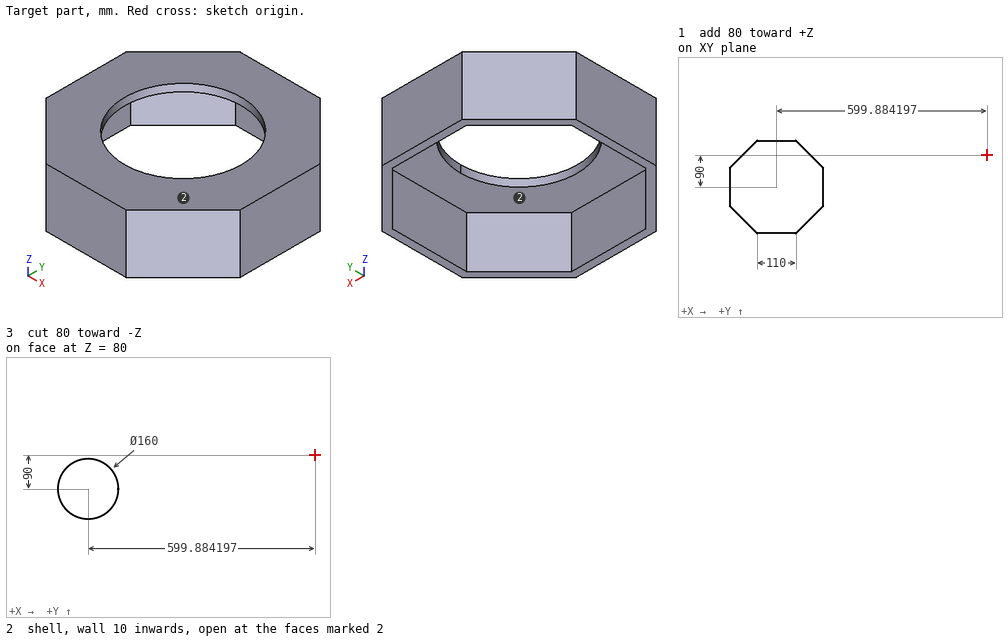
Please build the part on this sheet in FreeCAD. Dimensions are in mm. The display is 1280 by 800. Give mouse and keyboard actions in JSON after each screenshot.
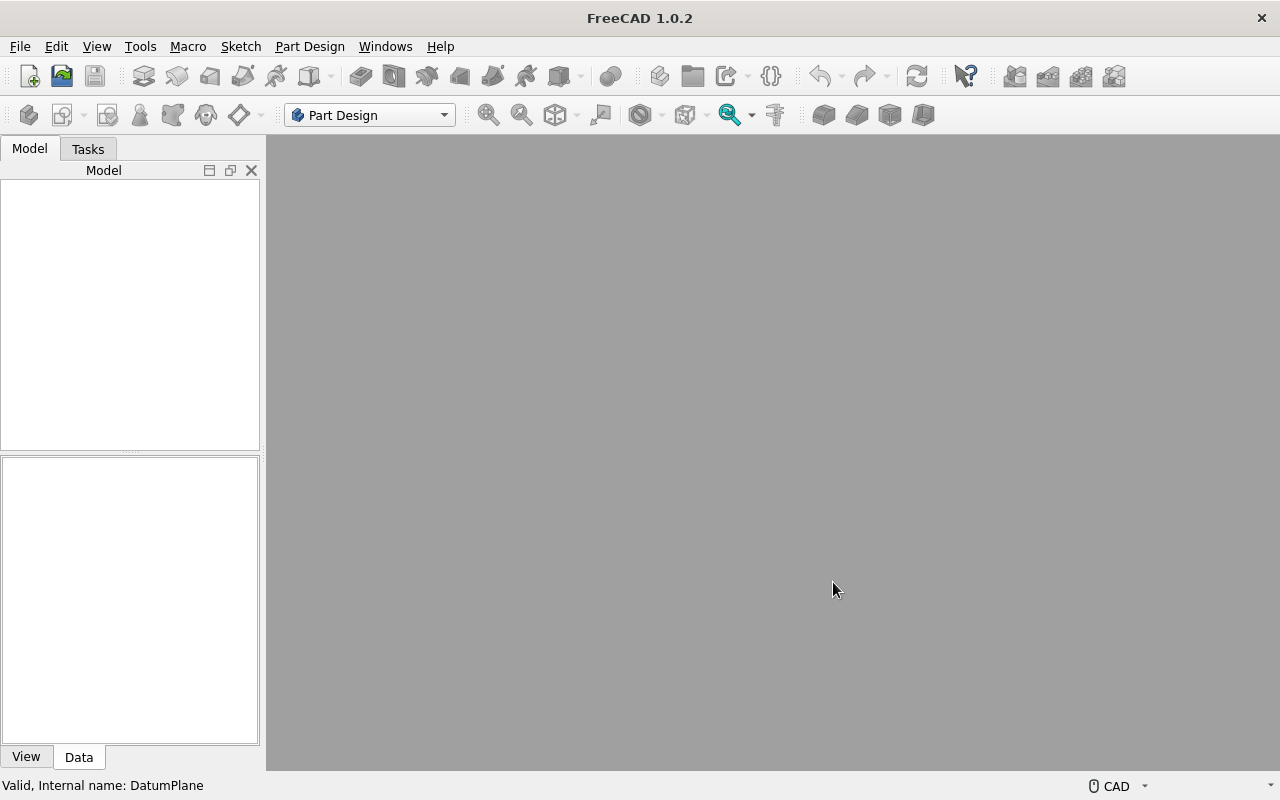
{"action": "key", "text": "ctrl+n"}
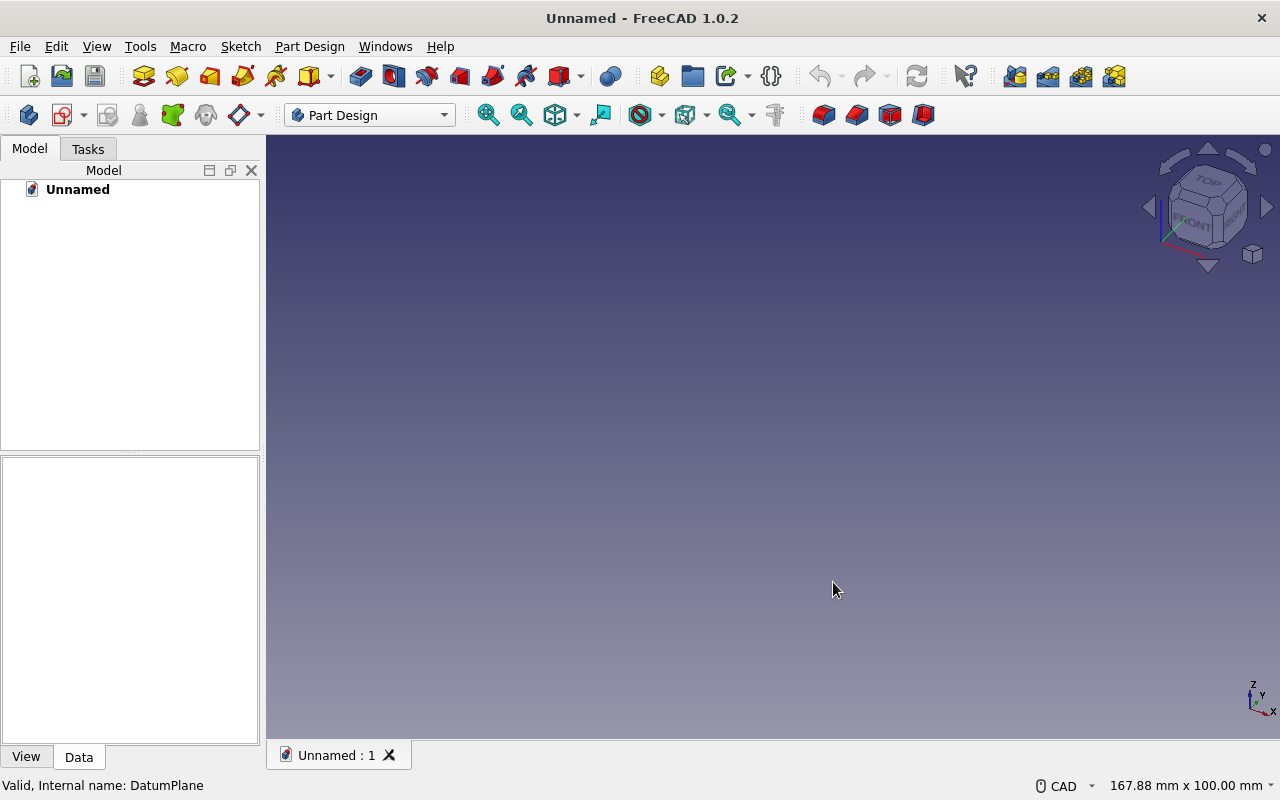
{"action": "left_click", "coordinate": [62, 116]}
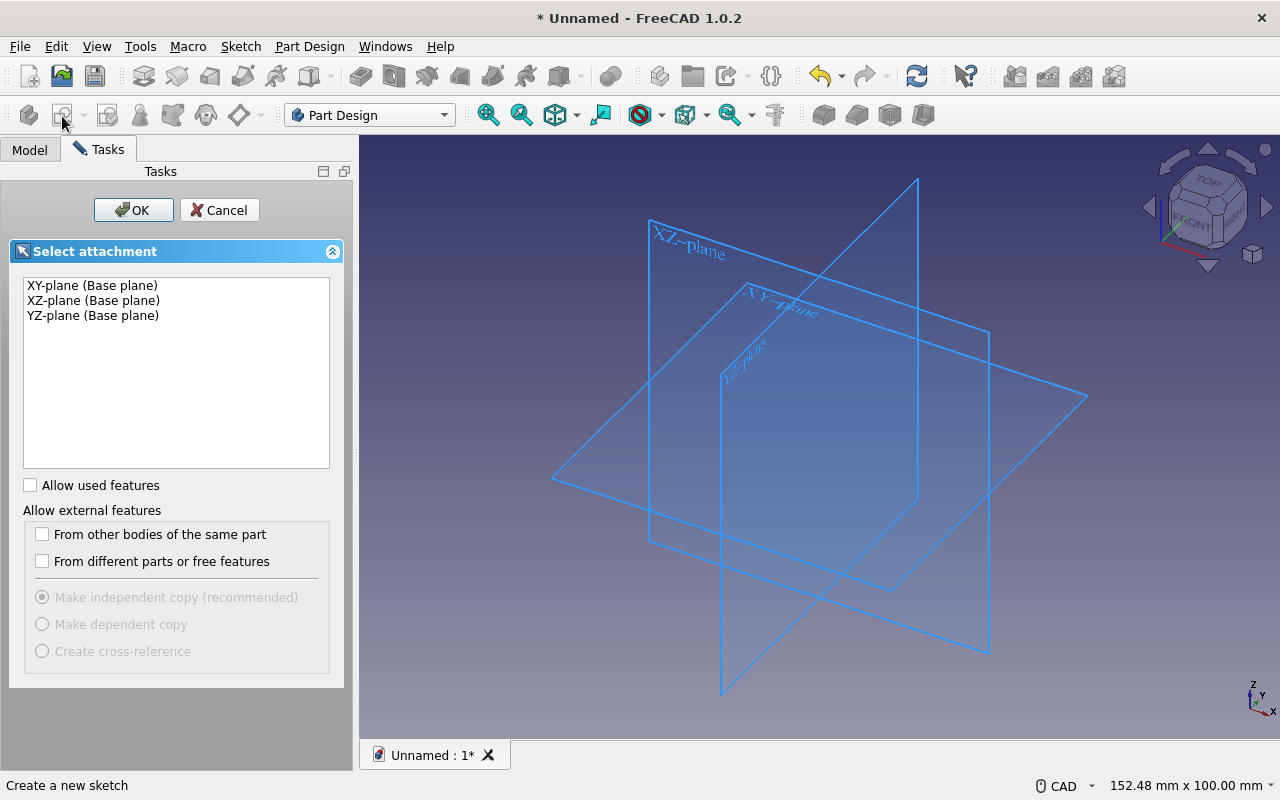
{"action": "left_click", "coordinate": [84, 286]}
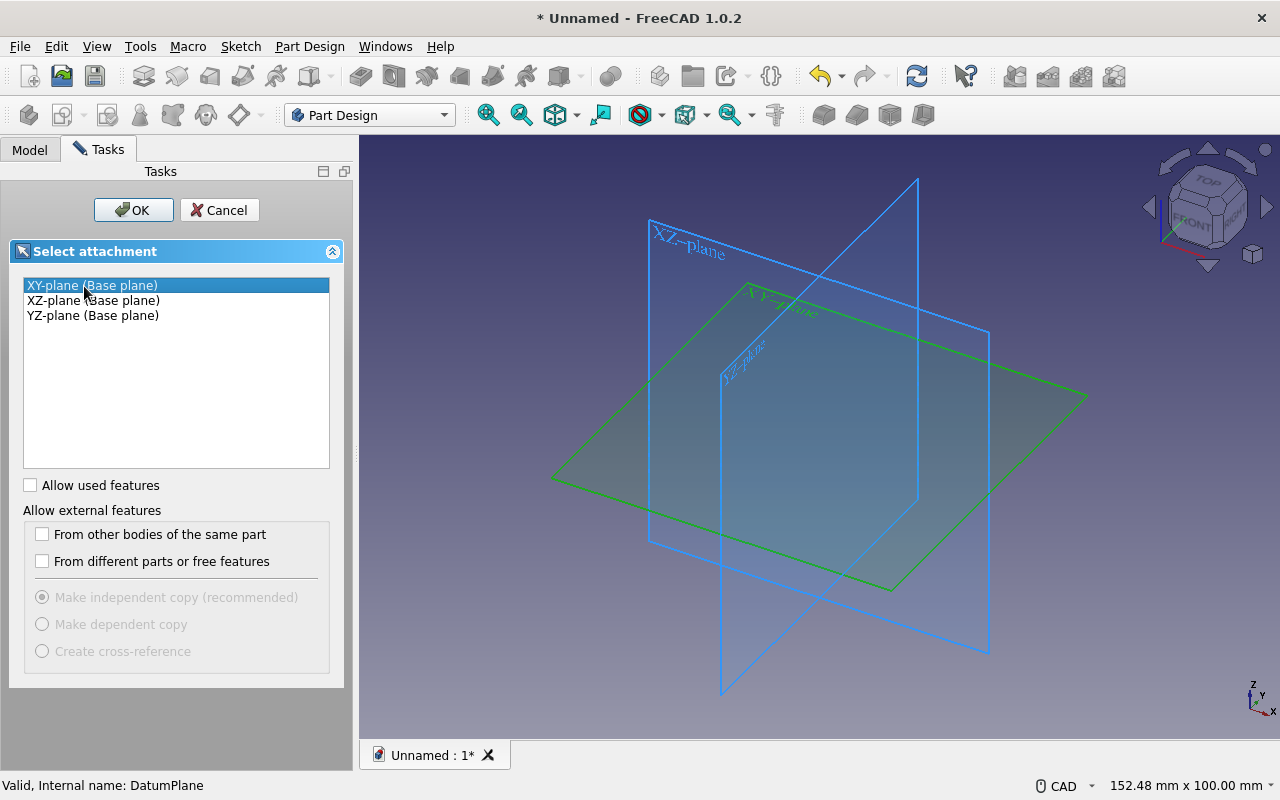
{"action": "left_click", "coordinate": [134, 210]}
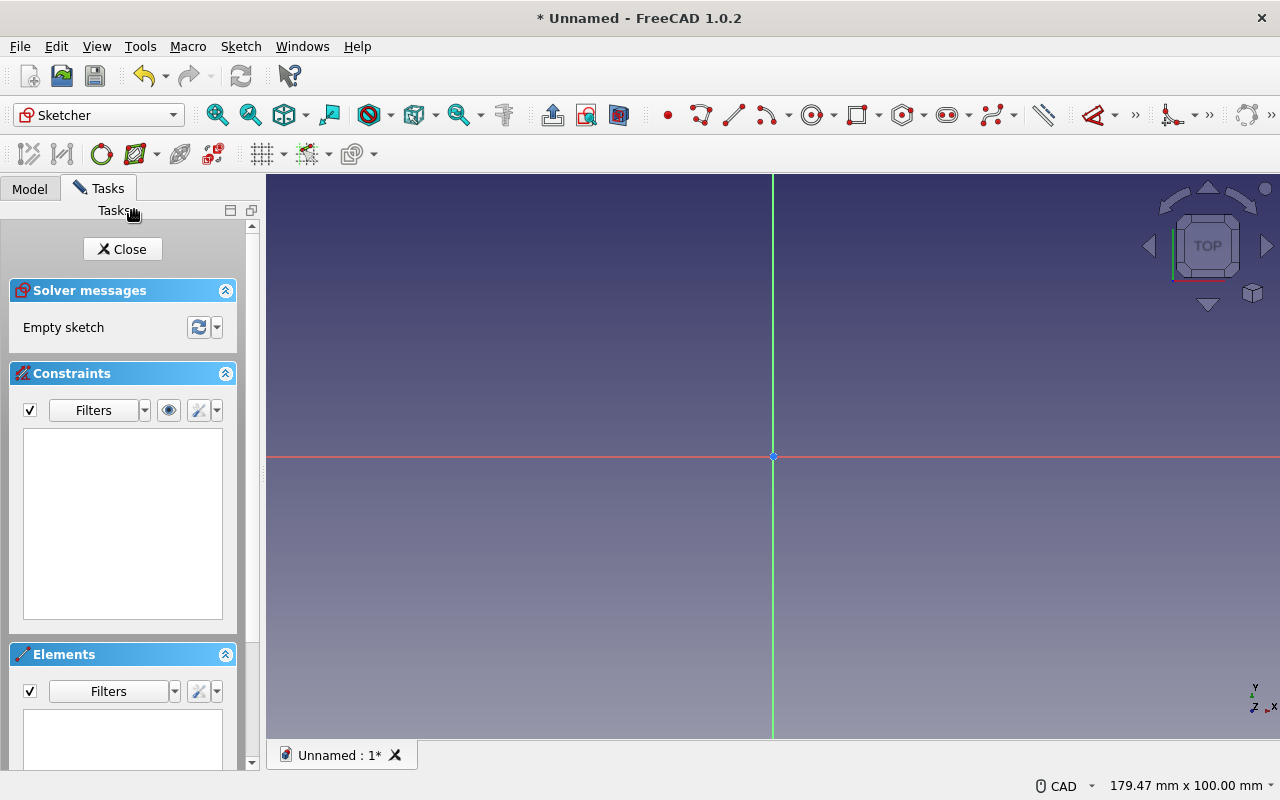
{"action": "scroll", "coordinate": [1115, 356], "scroll_direction": "down", "scroll_amount": 9}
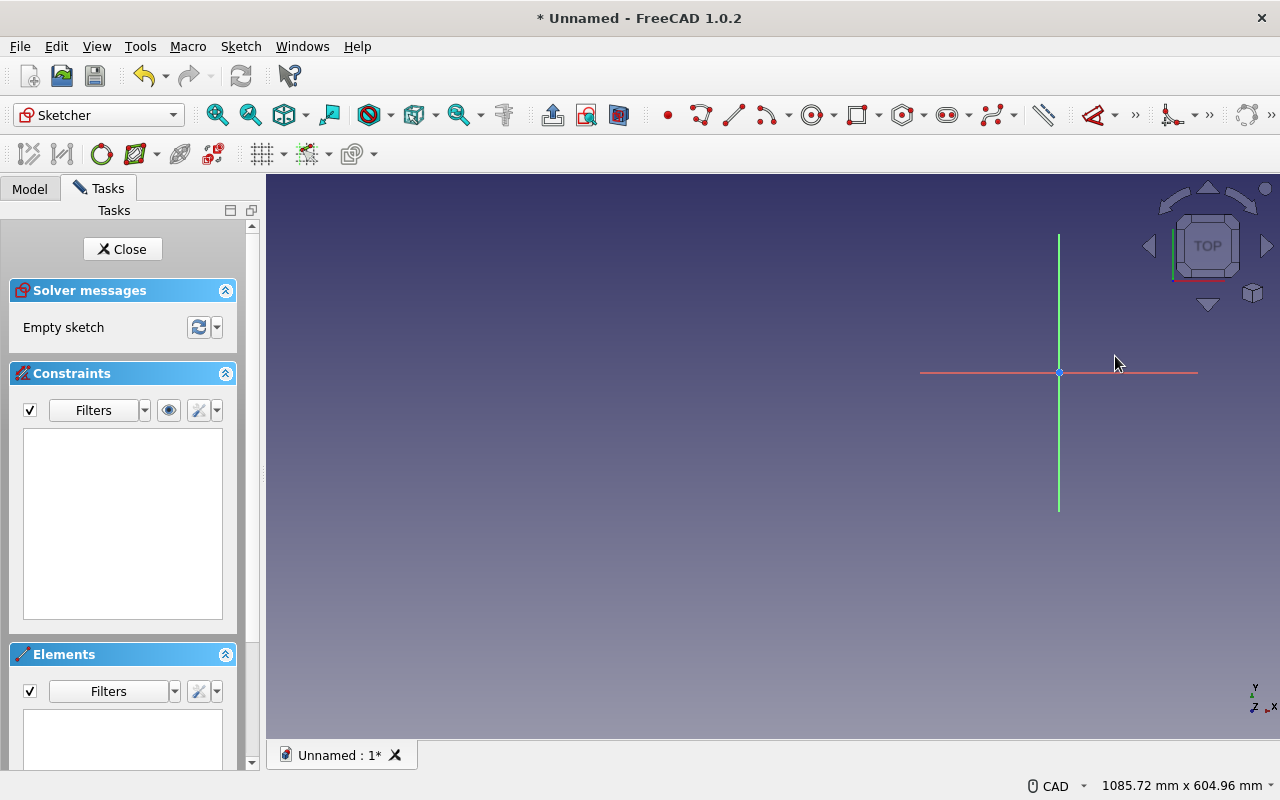
{"action": "scroll", "coordinate": [294, 458], "scroll_direction": "up", "scroll_amount": 2}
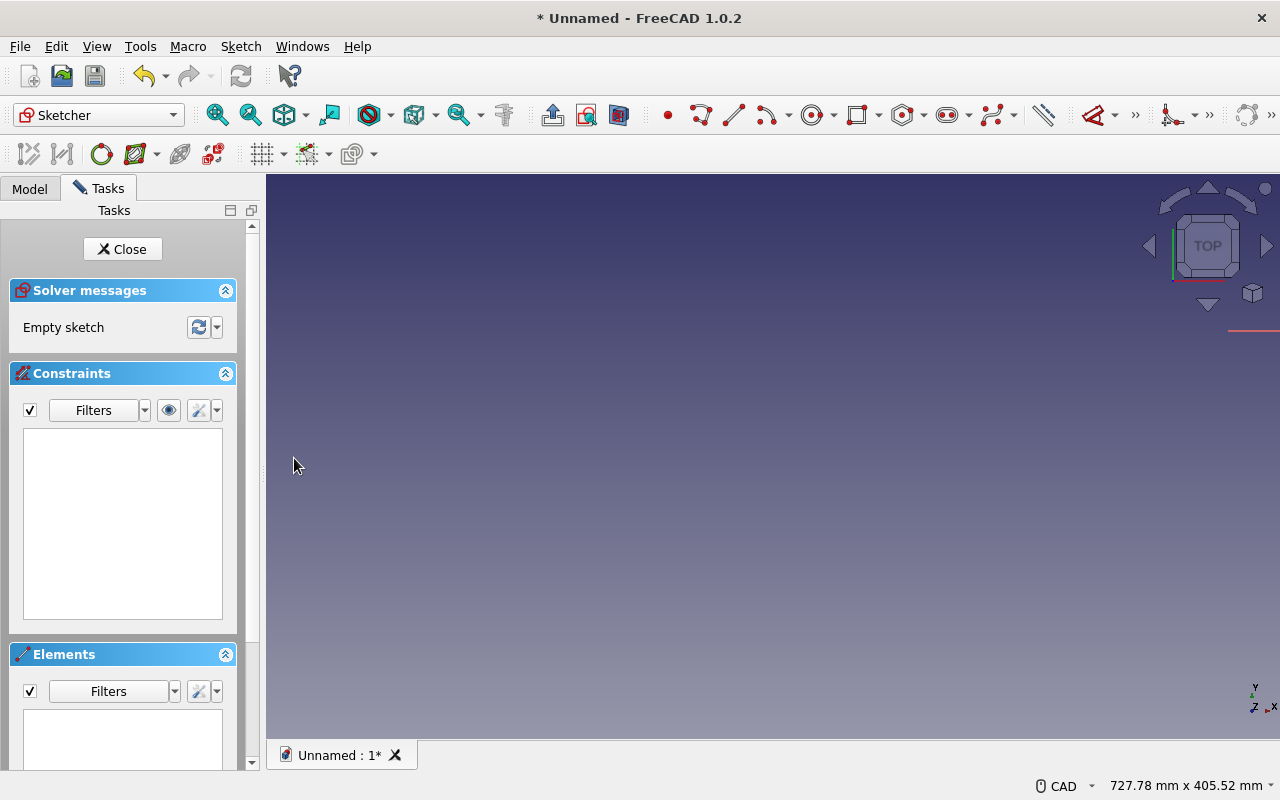
{"action": "key", "text": "g p 8"}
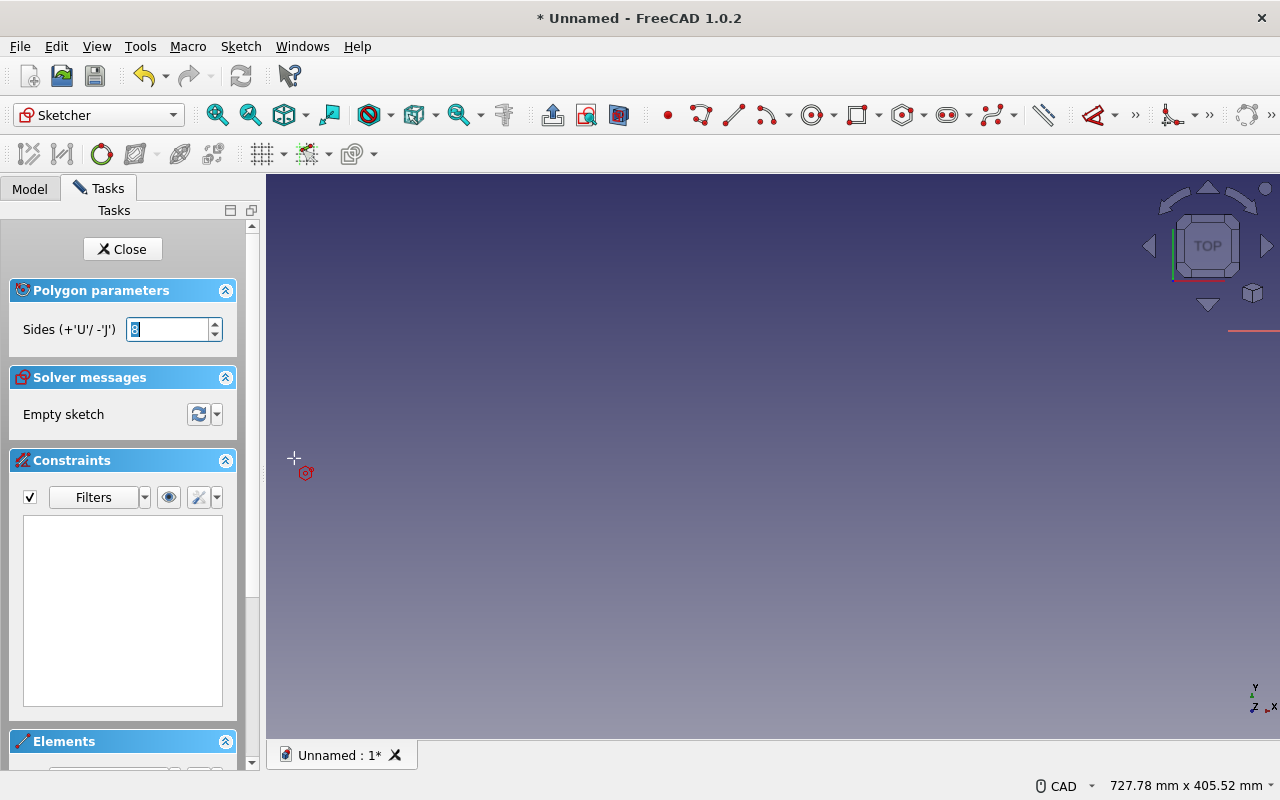
{"action": "left_click", "coordinate": [600, 456]}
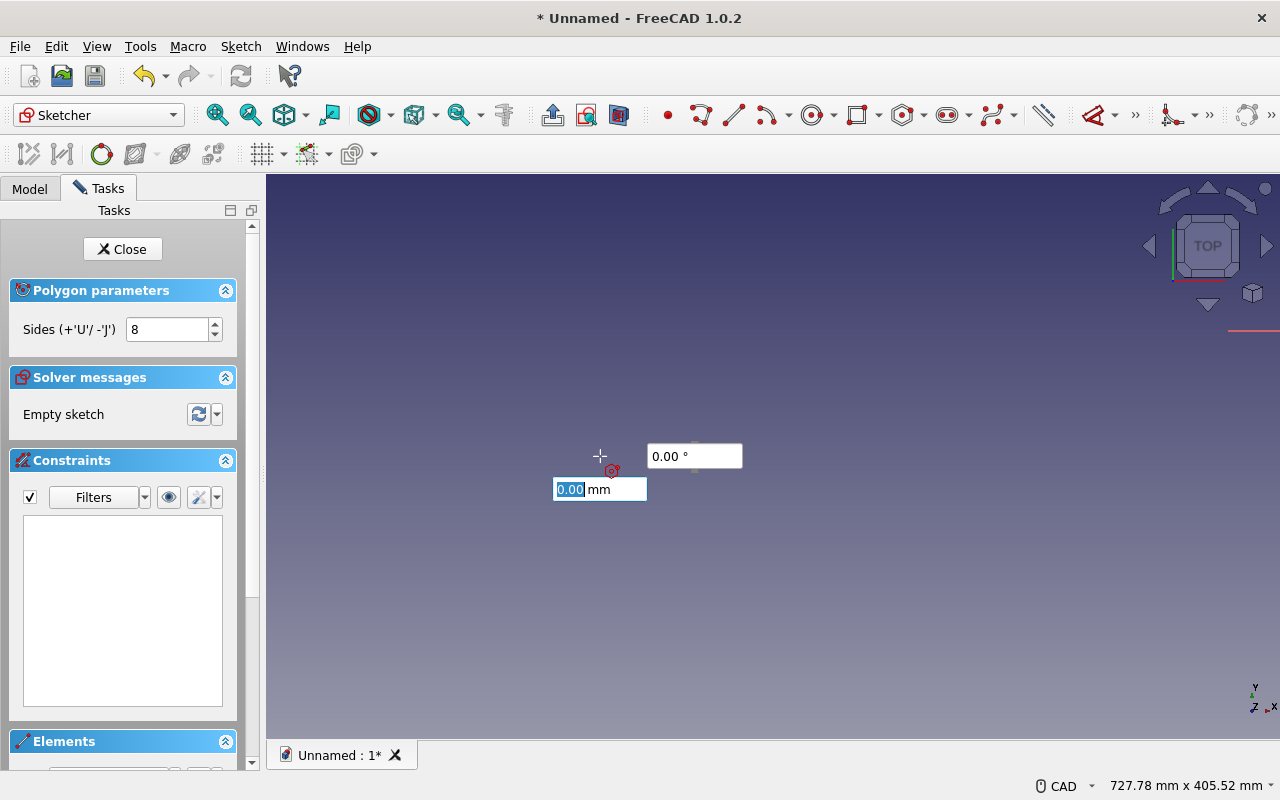
{"action": "left_click", "coordinate": [523, 641]}
{"action": "right_click", "coordinate": [523, 641]}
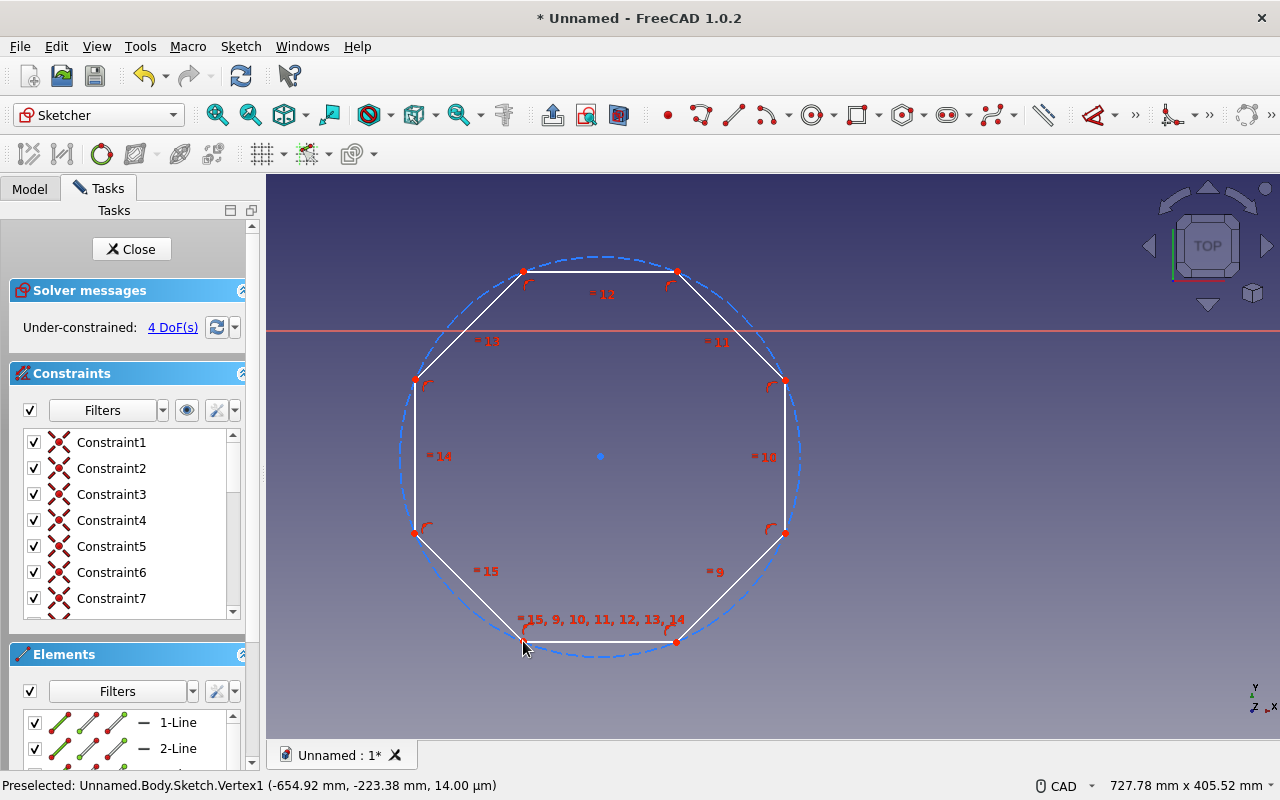
{"action": "left_click", "coordinate": [569, 642]}